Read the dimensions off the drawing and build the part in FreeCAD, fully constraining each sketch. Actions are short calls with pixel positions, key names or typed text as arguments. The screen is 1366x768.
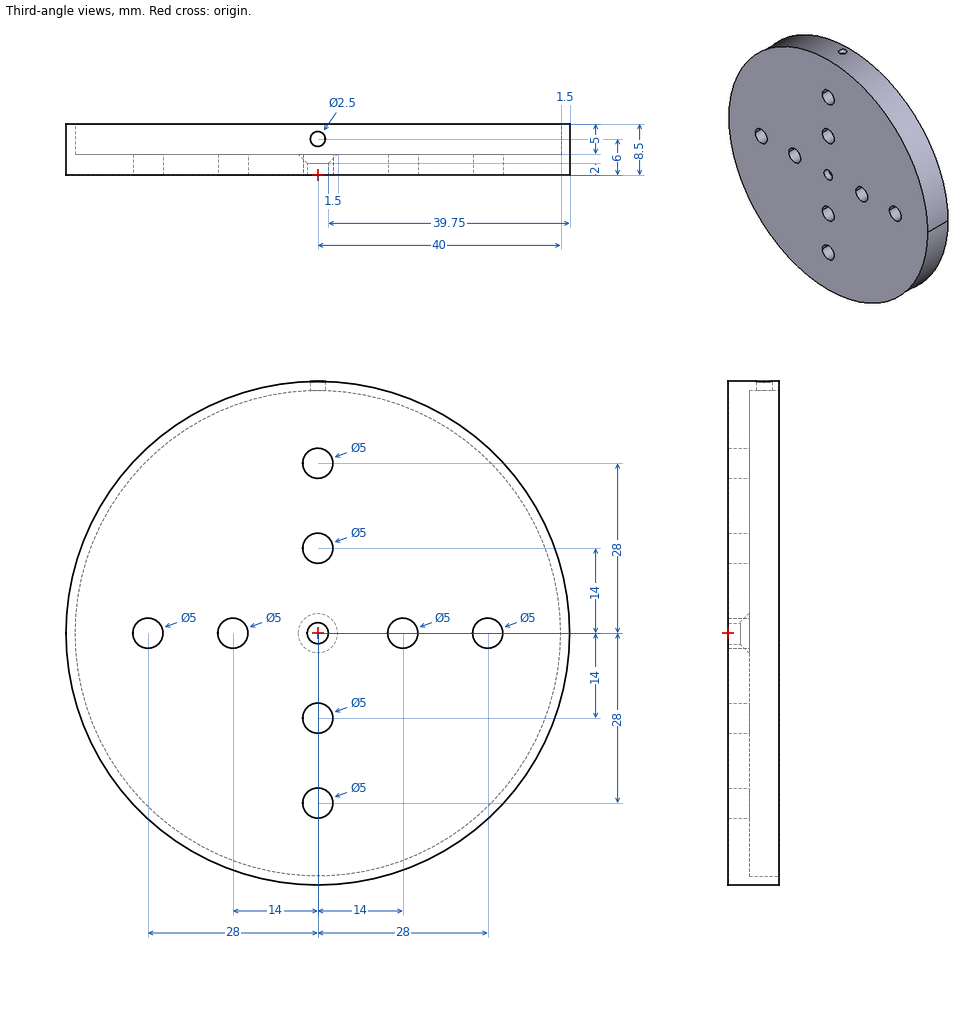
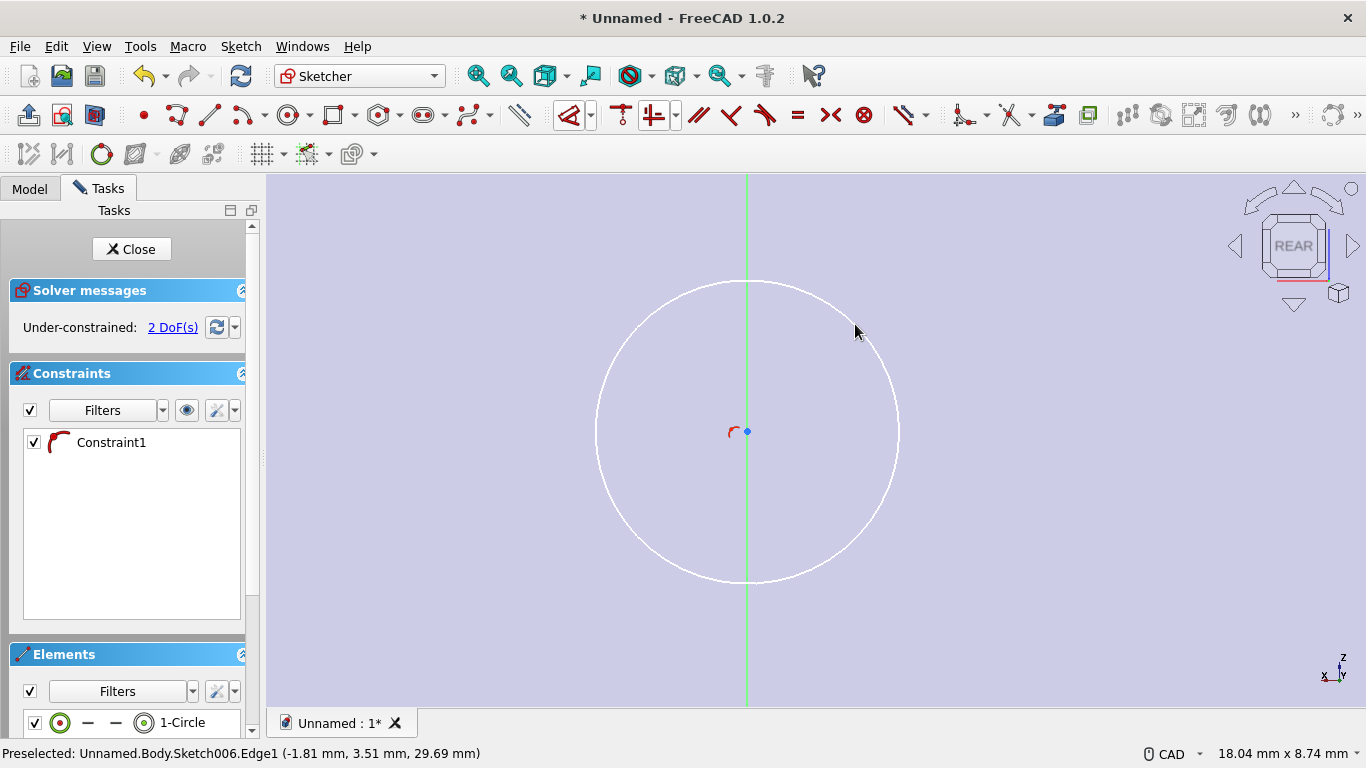
click(854, 324)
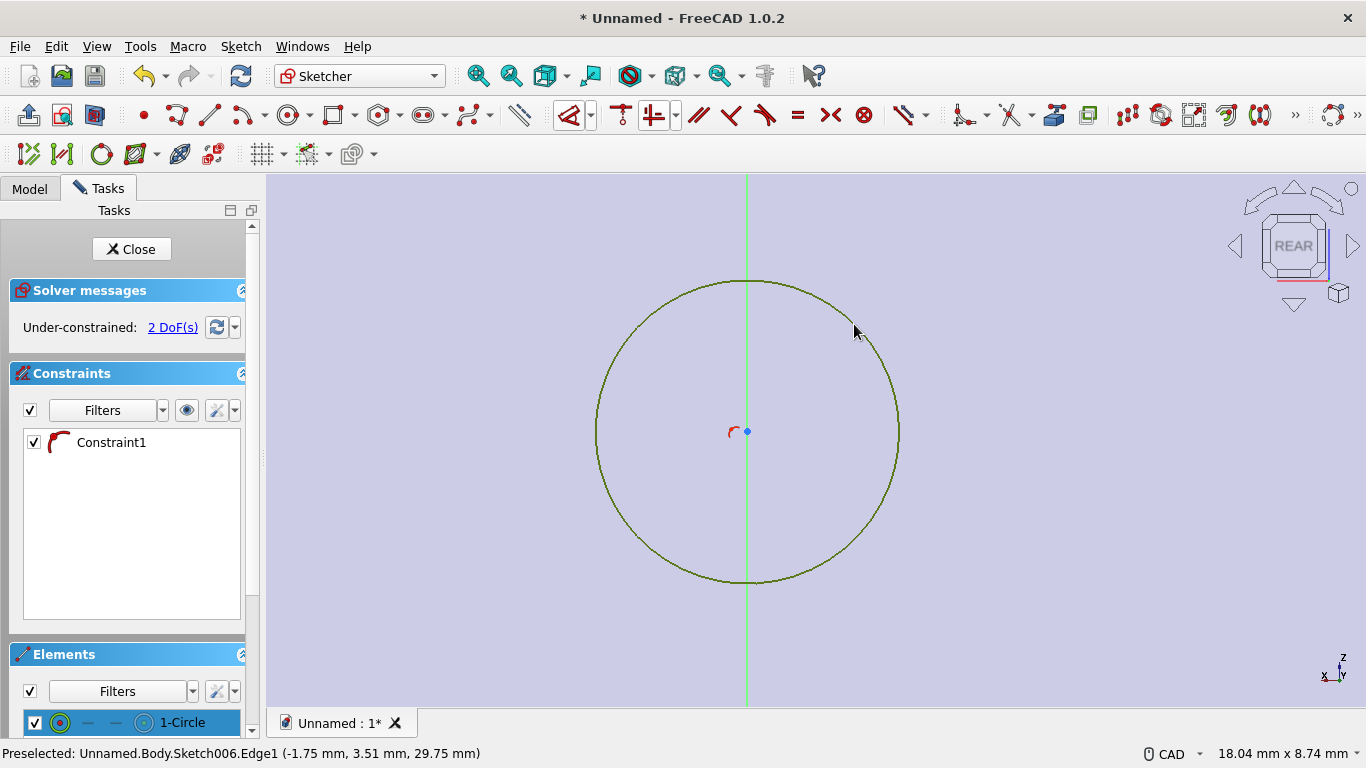
click(590, 116)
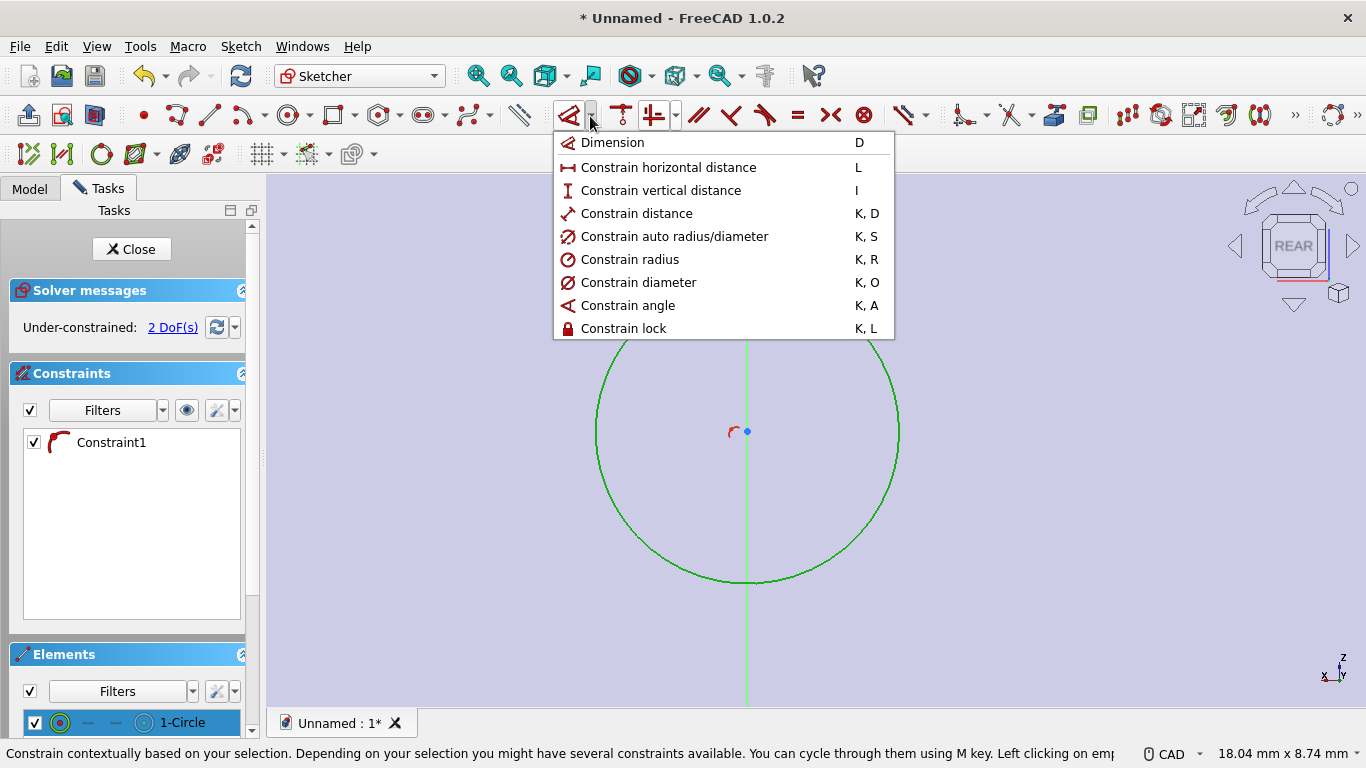
click(724, 282)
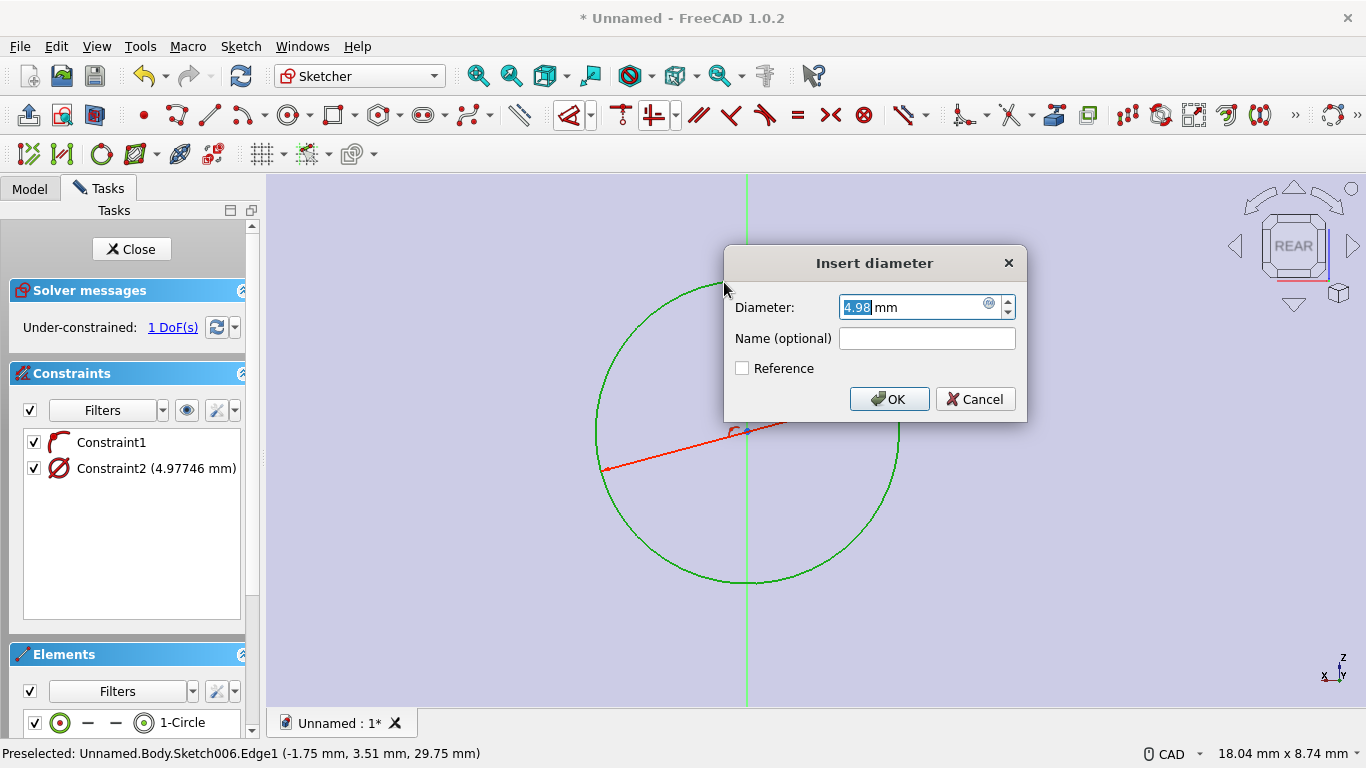
text(5)
key(Return)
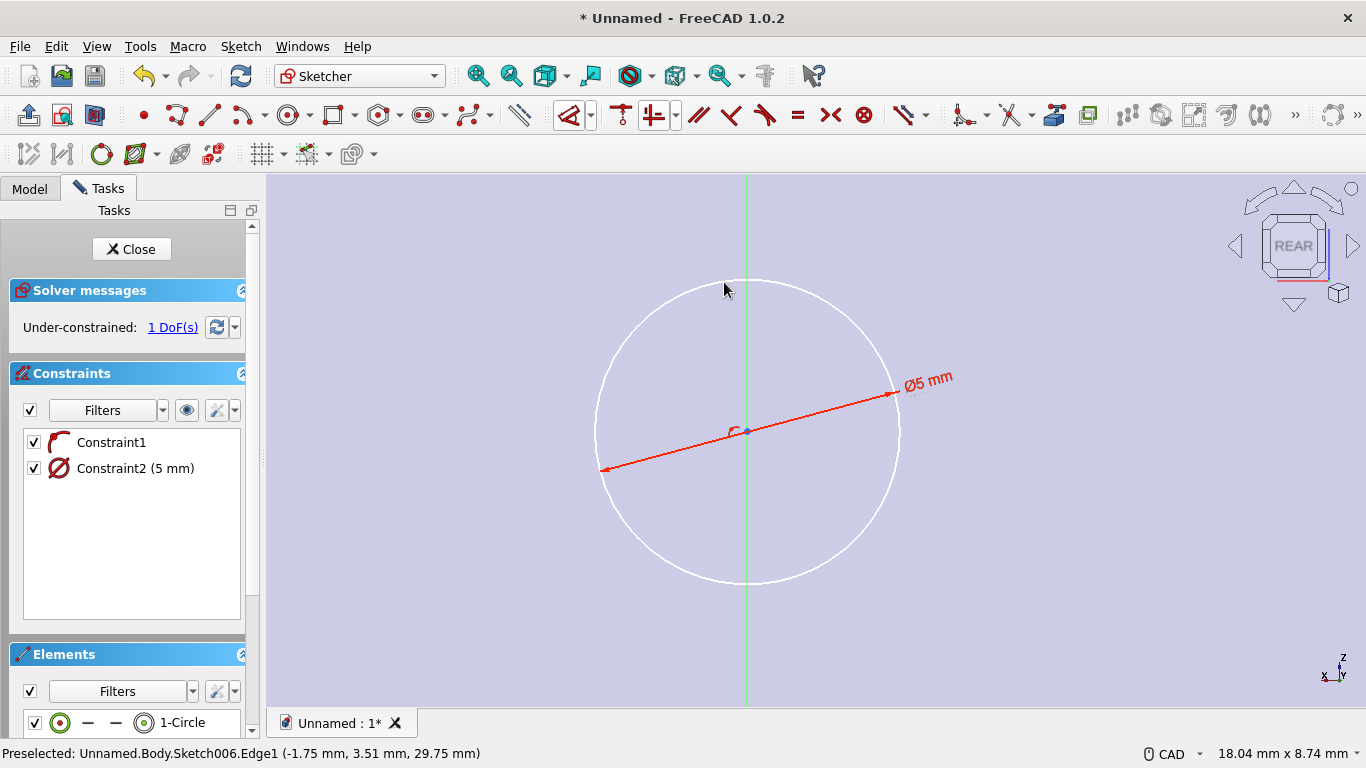
click(747, 432)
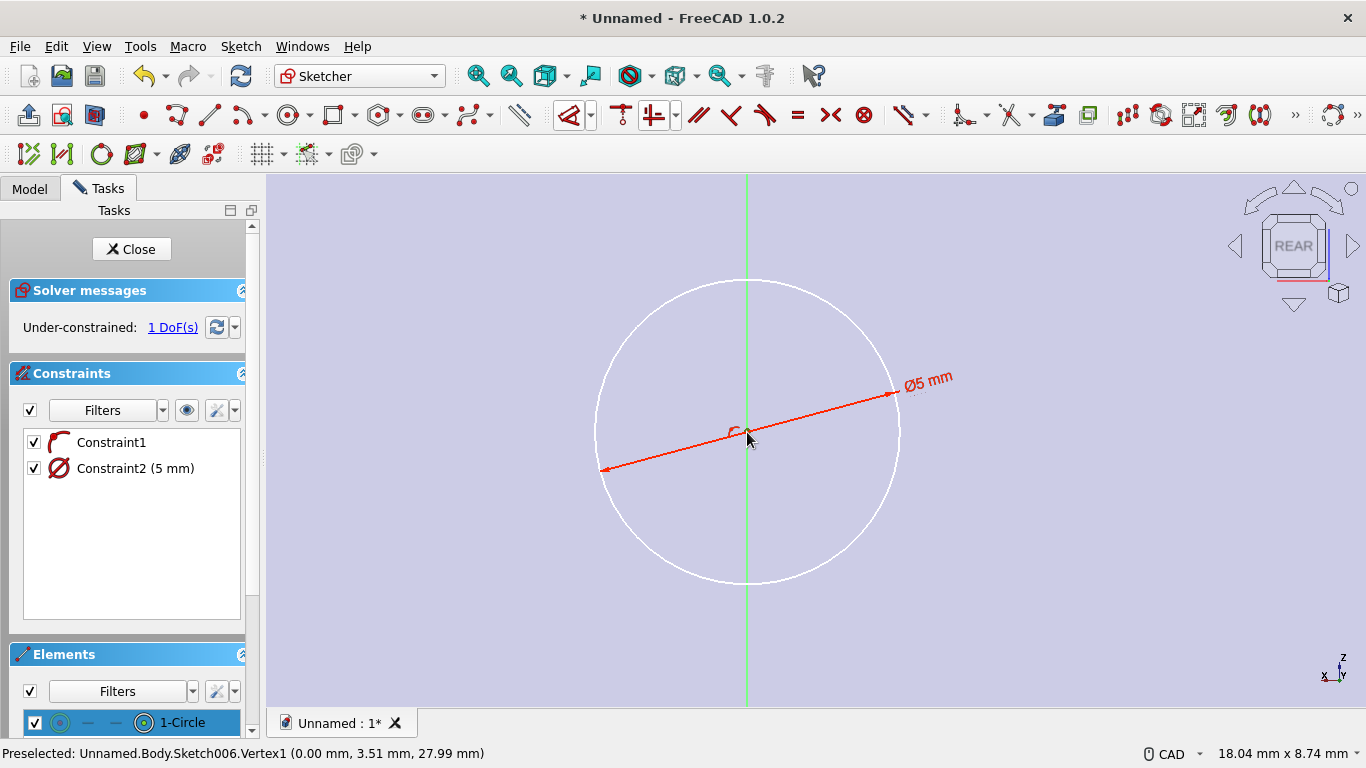
click(590, 116)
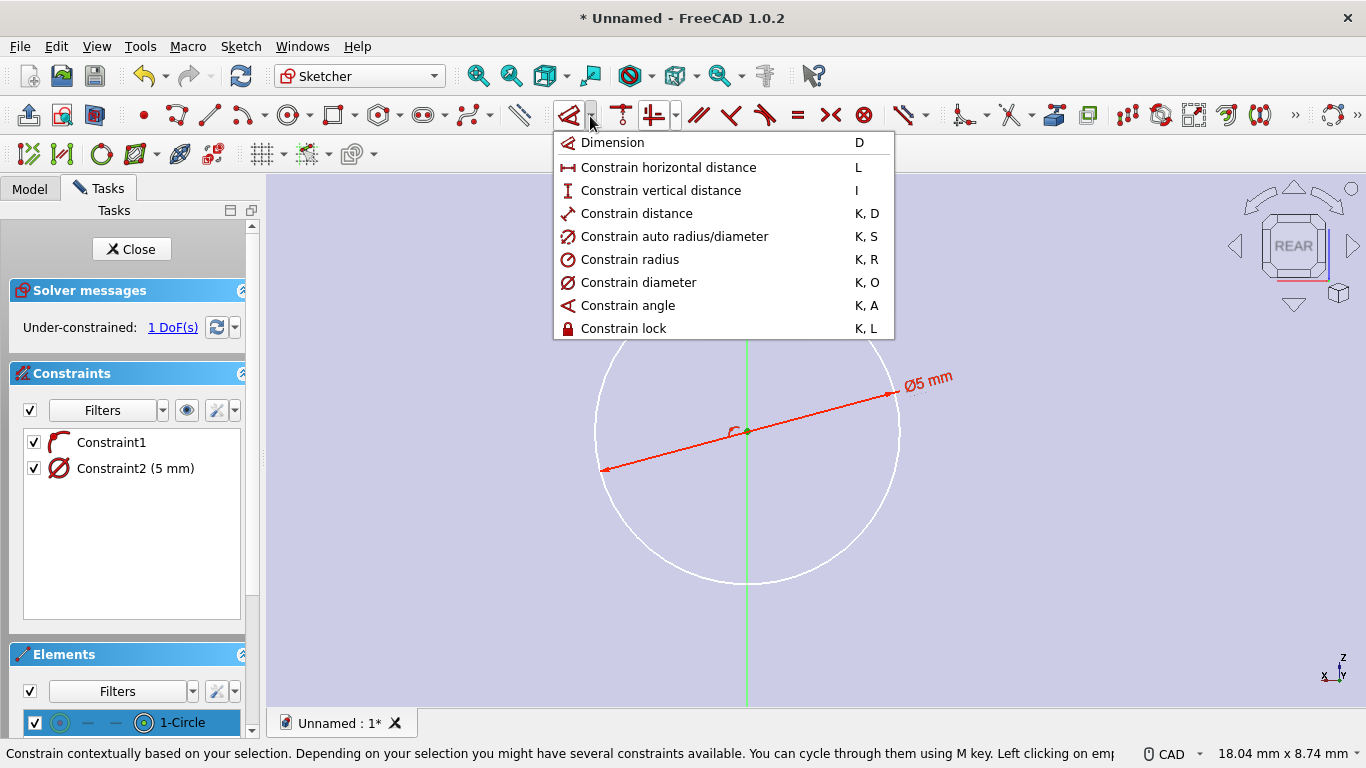
click(724, 190)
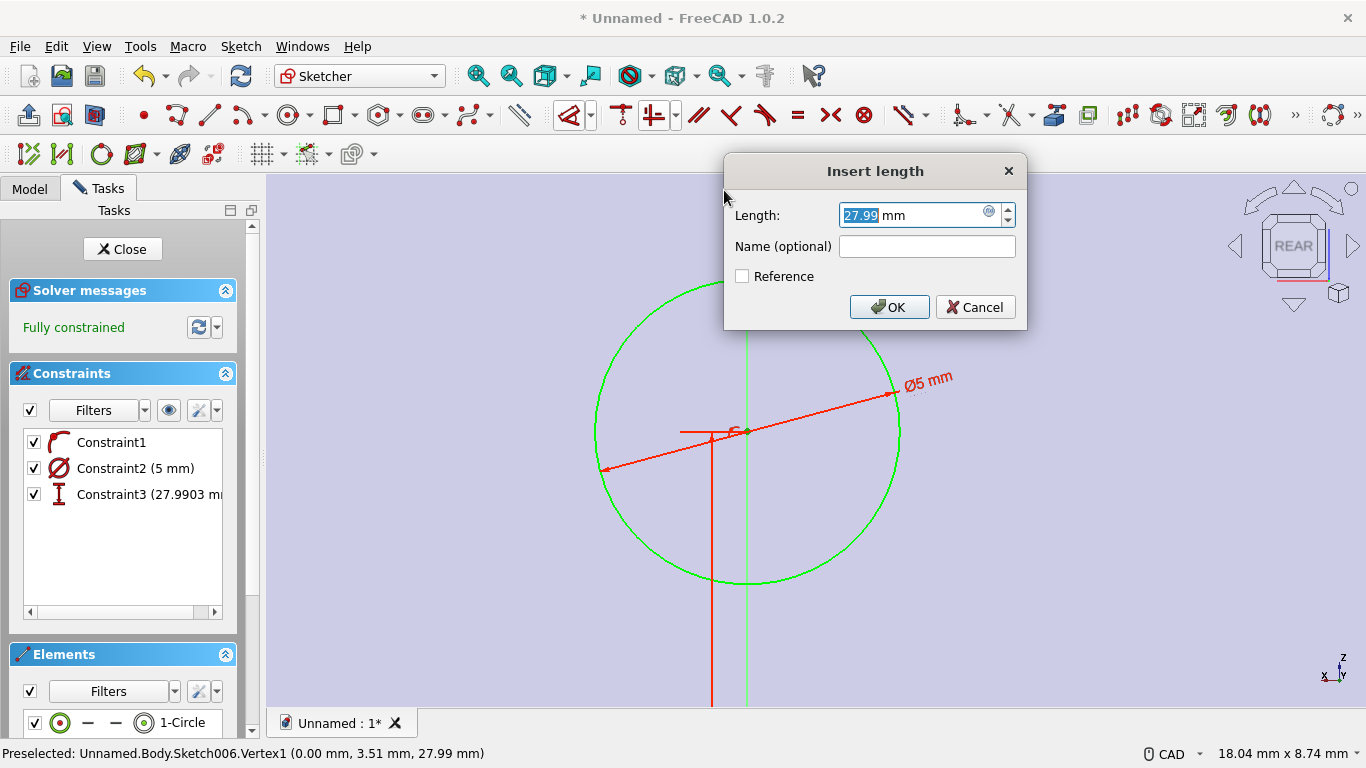
text(28)
key(Return)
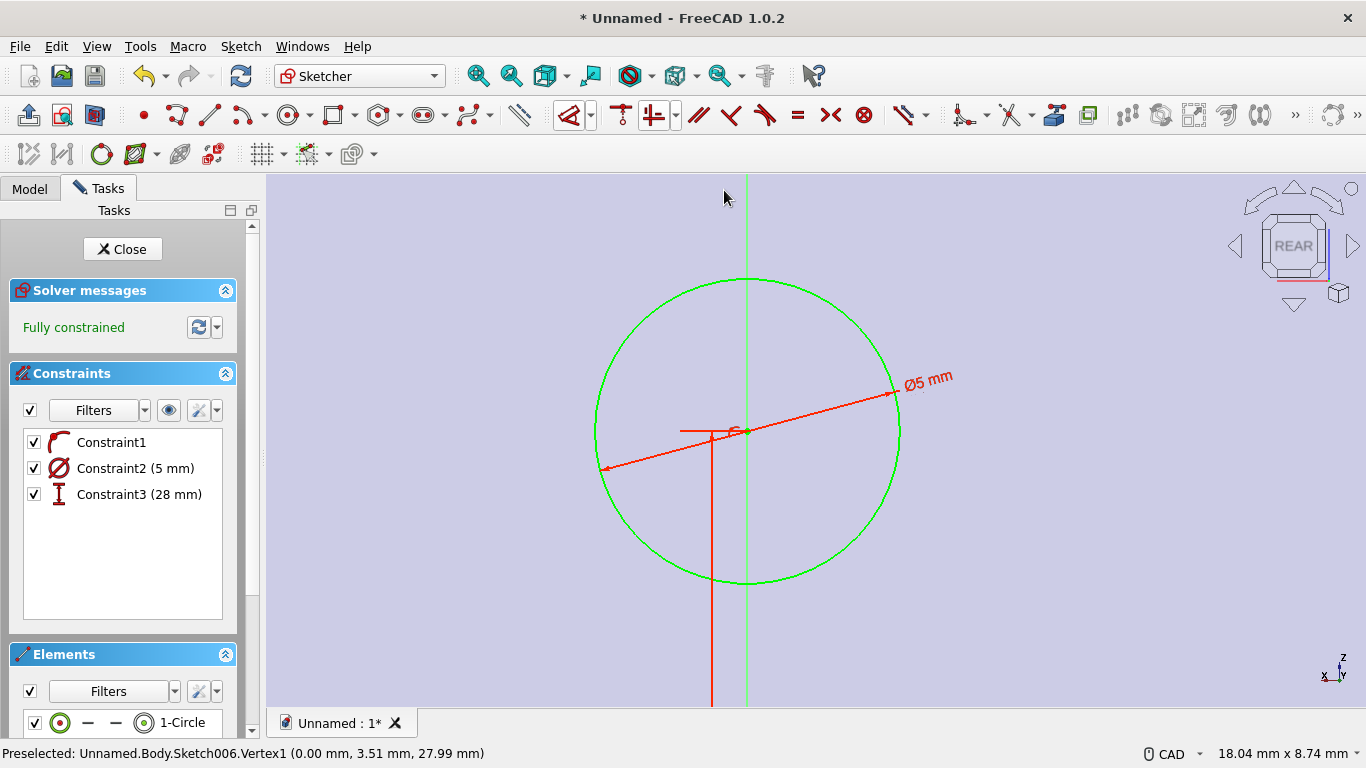
click(123, 249)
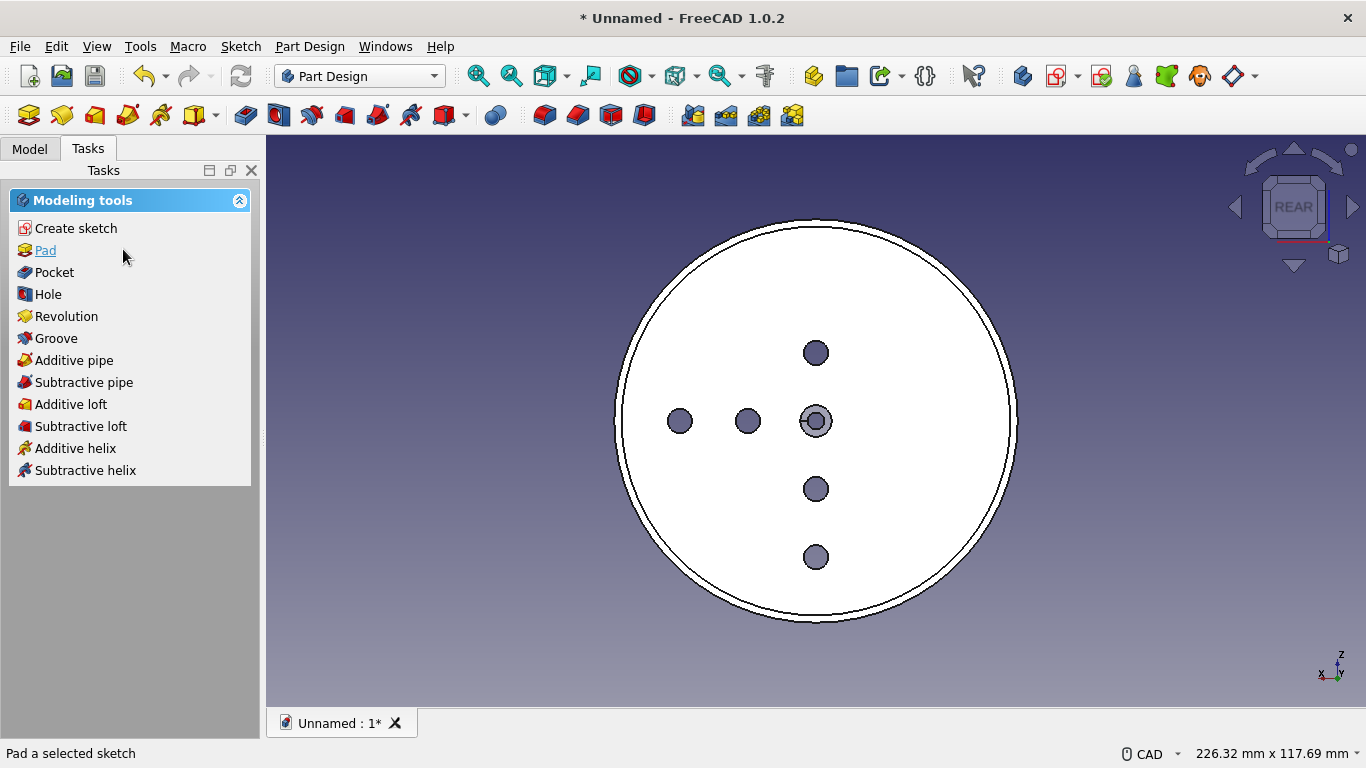
click(246, 116)